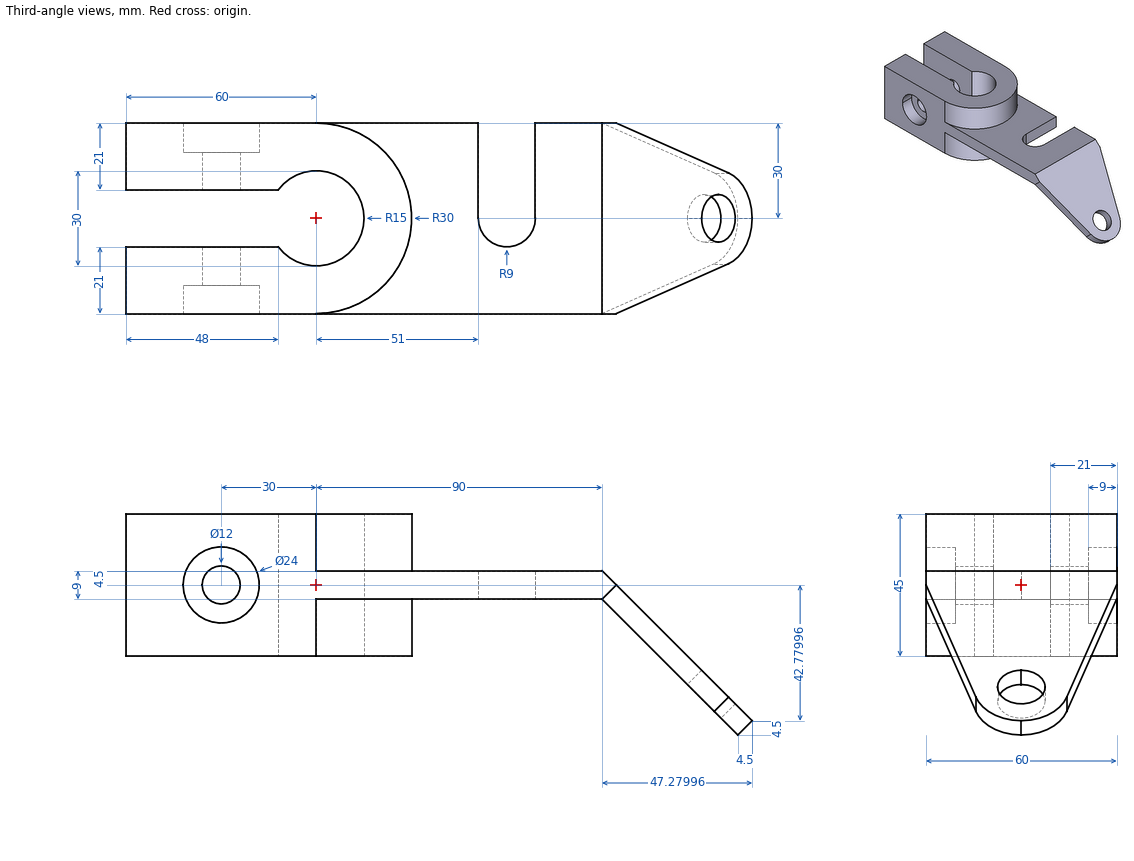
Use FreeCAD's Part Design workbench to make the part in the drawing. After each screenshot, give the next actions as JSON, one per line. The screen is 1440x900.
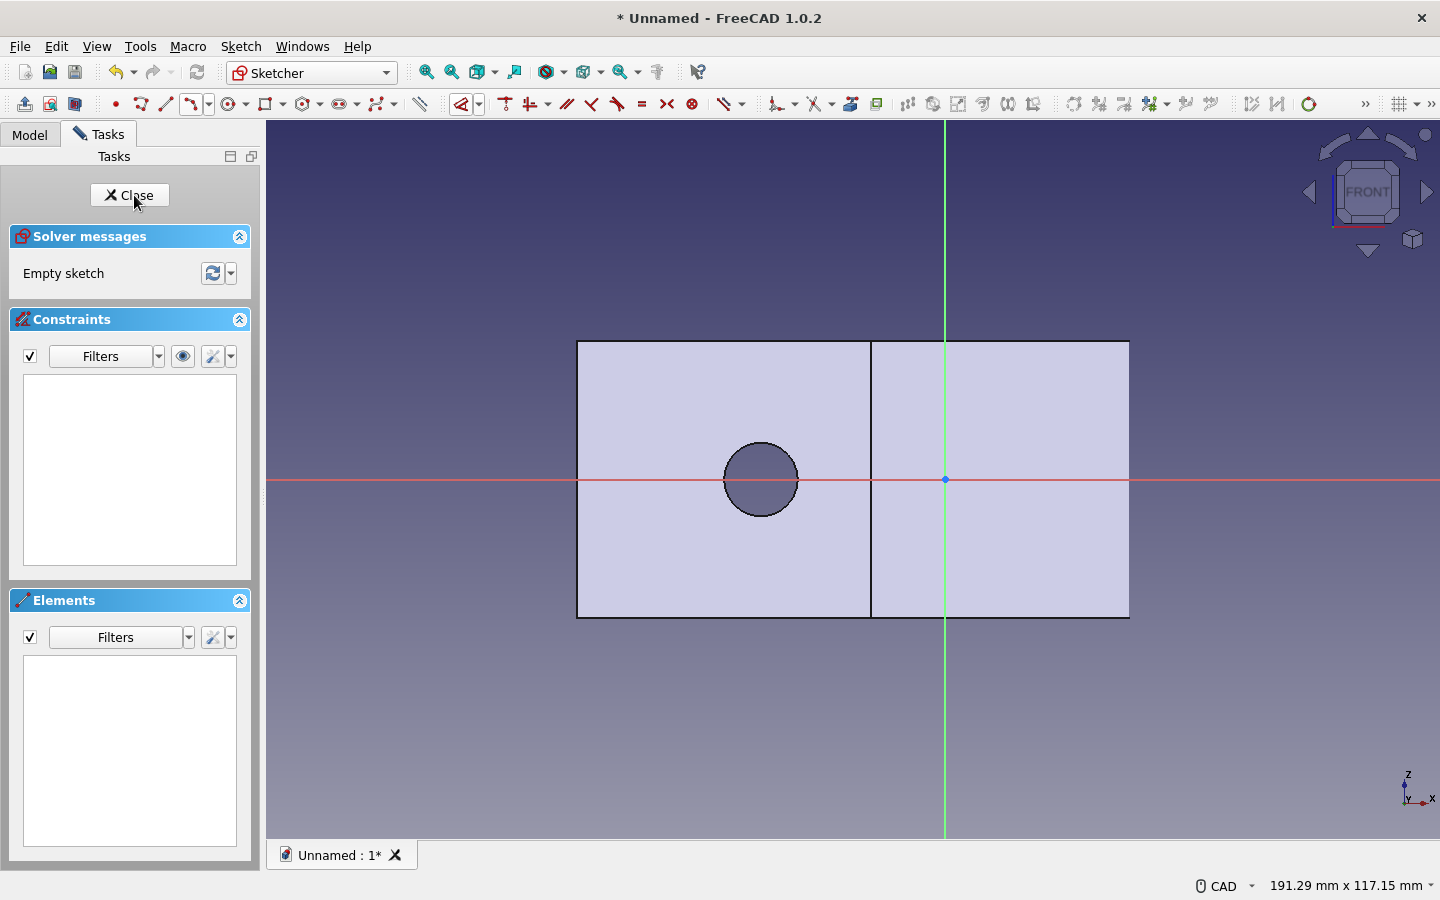
{"action": "scroll", "coordinate": [294, 320], "scroll_direction": "down", "scroll_amount": 3}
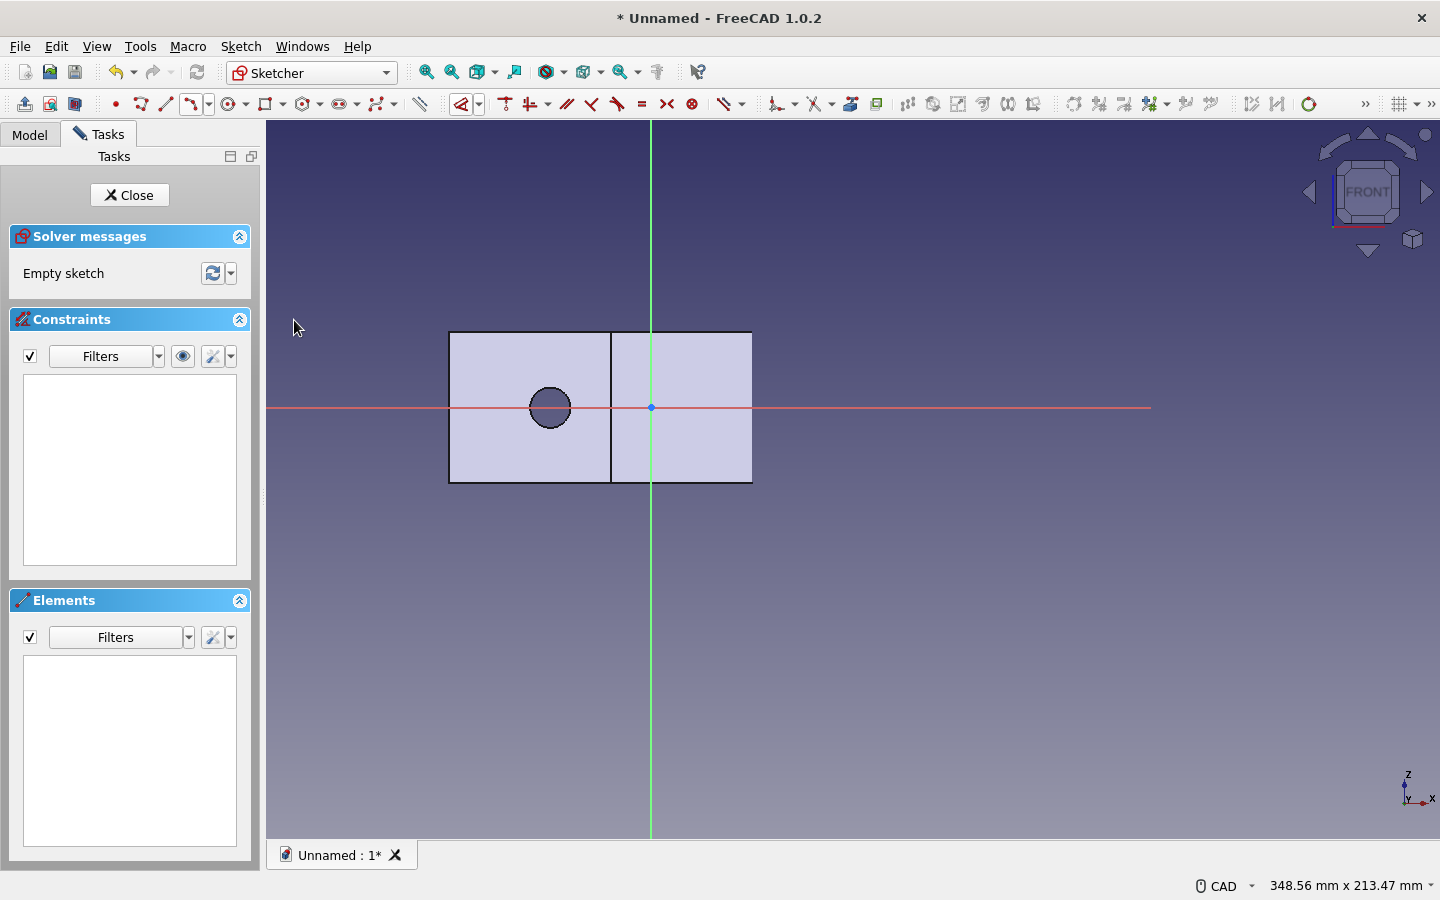
{"action": "scroll", "coordinate": [1082, 480], "scroll_direction": "up", "scroll_amount": 2}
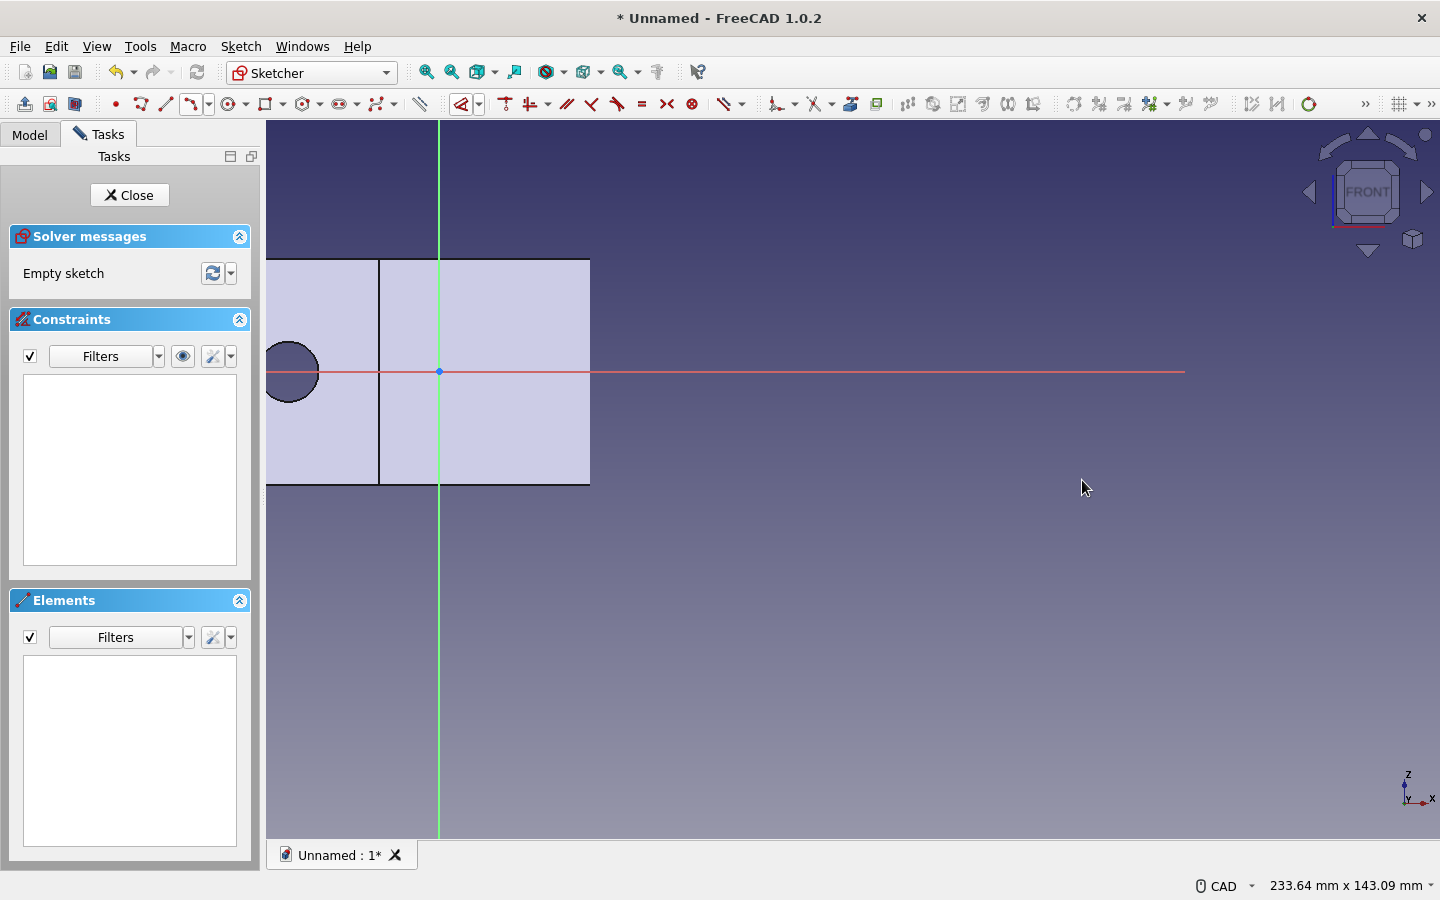
{"action": "left_click", "coordinate": [141, 104]}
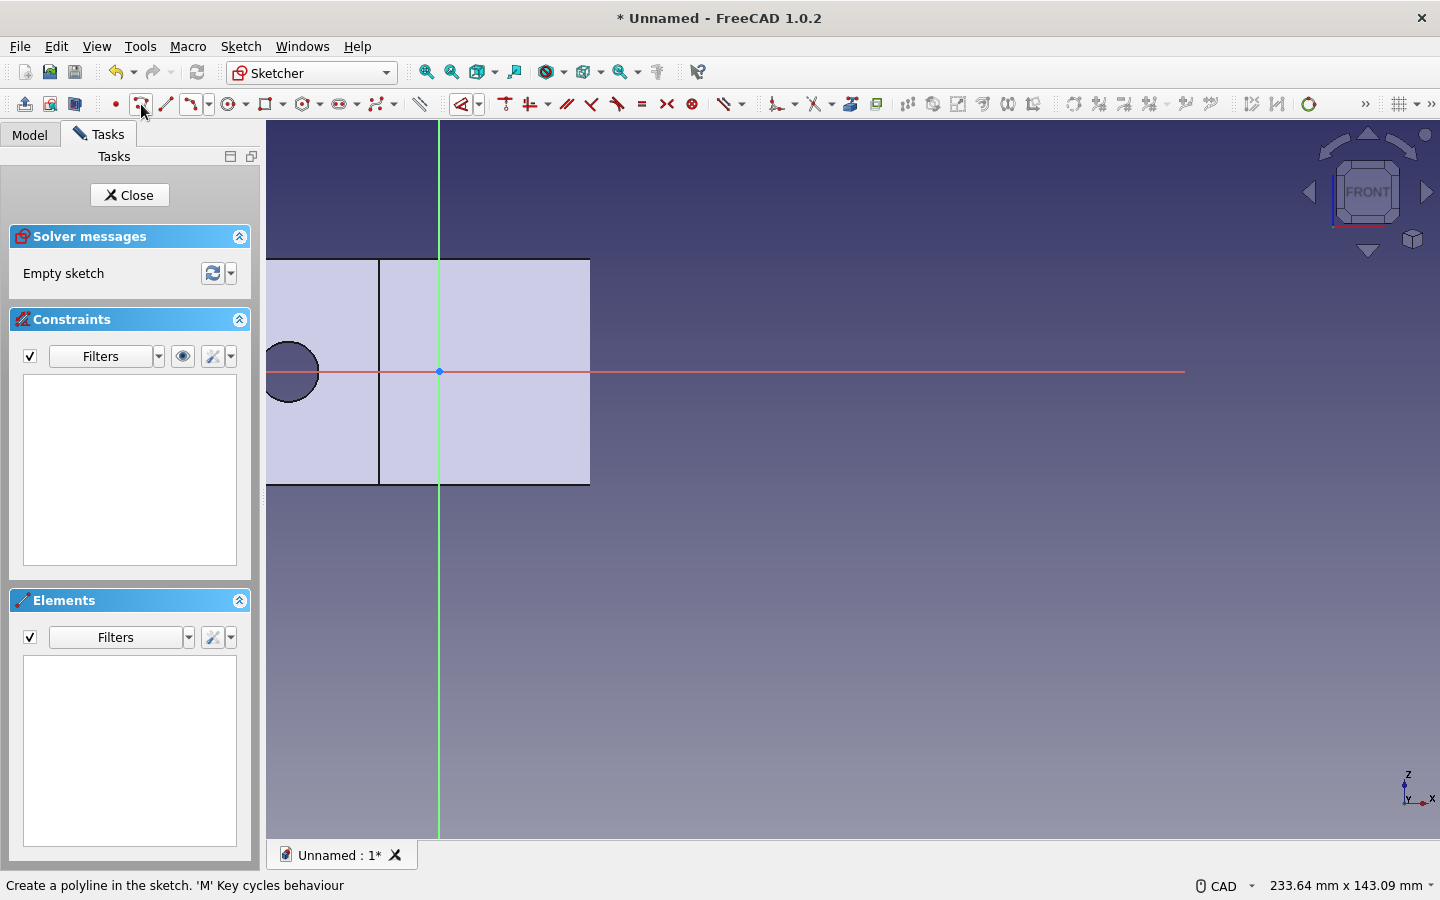
{"action": "left_click", "coordinate": [439, 349]}
{"action": "left_click", "coordinate": [891, 349]}
{"action": "left_click", "coordinate": [1129, 587]}
{"action": "left_click", "coordinate": [1106, 609]}
{"action": "left_click", "coordinate": [891, 394]}
{"action": "left_click", "coordinate": [448, 394]}
{"action": "left_click", "coordinate": [439, 350]}
{"action": "key", "text": "Escape"}
{"action": "key", "text": "Escape"}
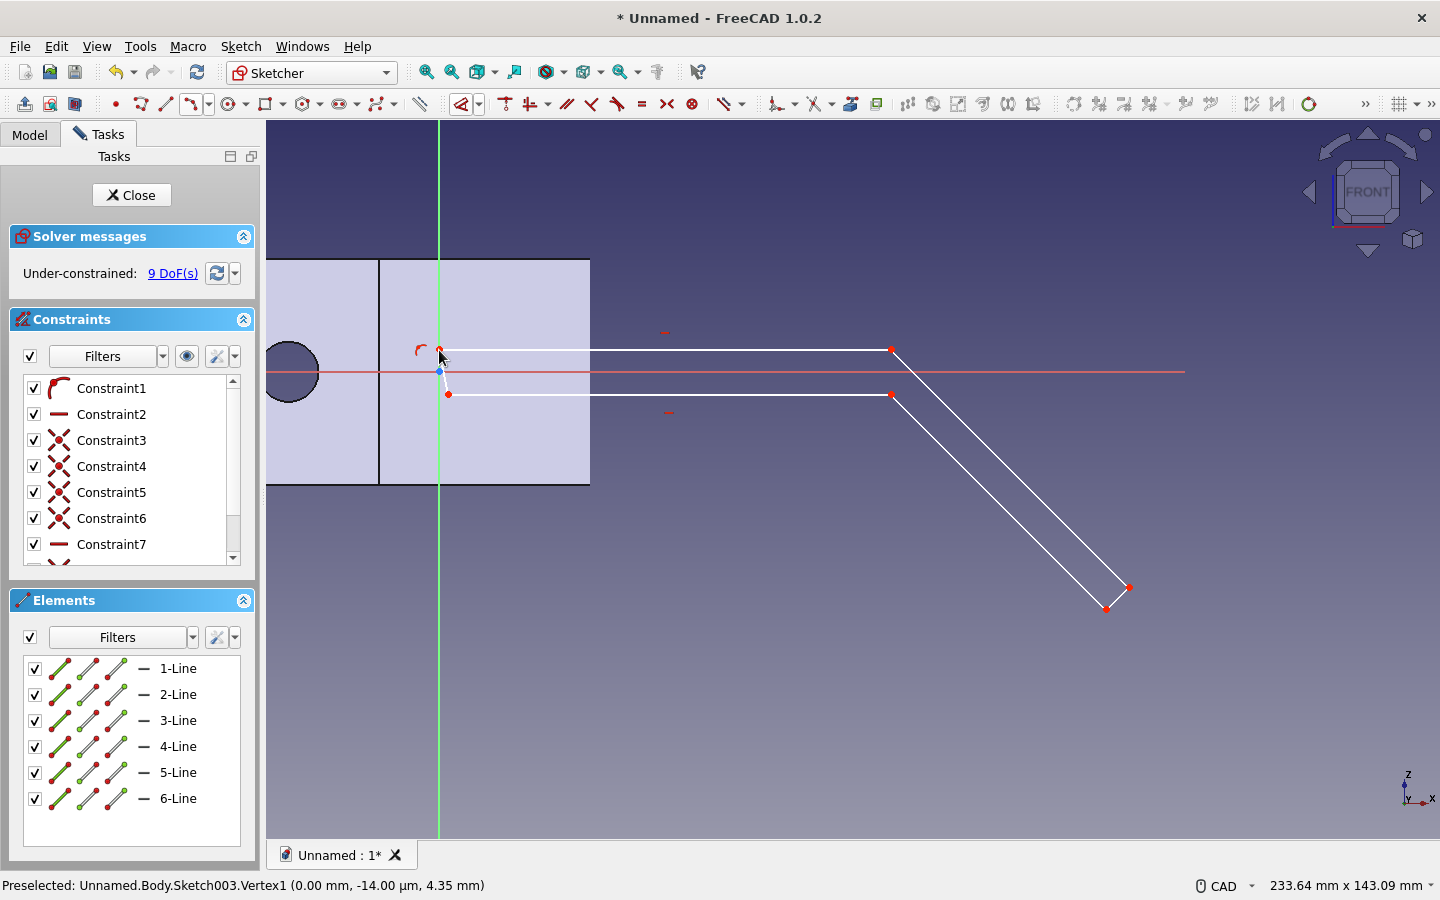
{"action": "left_click", "coordinate": [441, 359]}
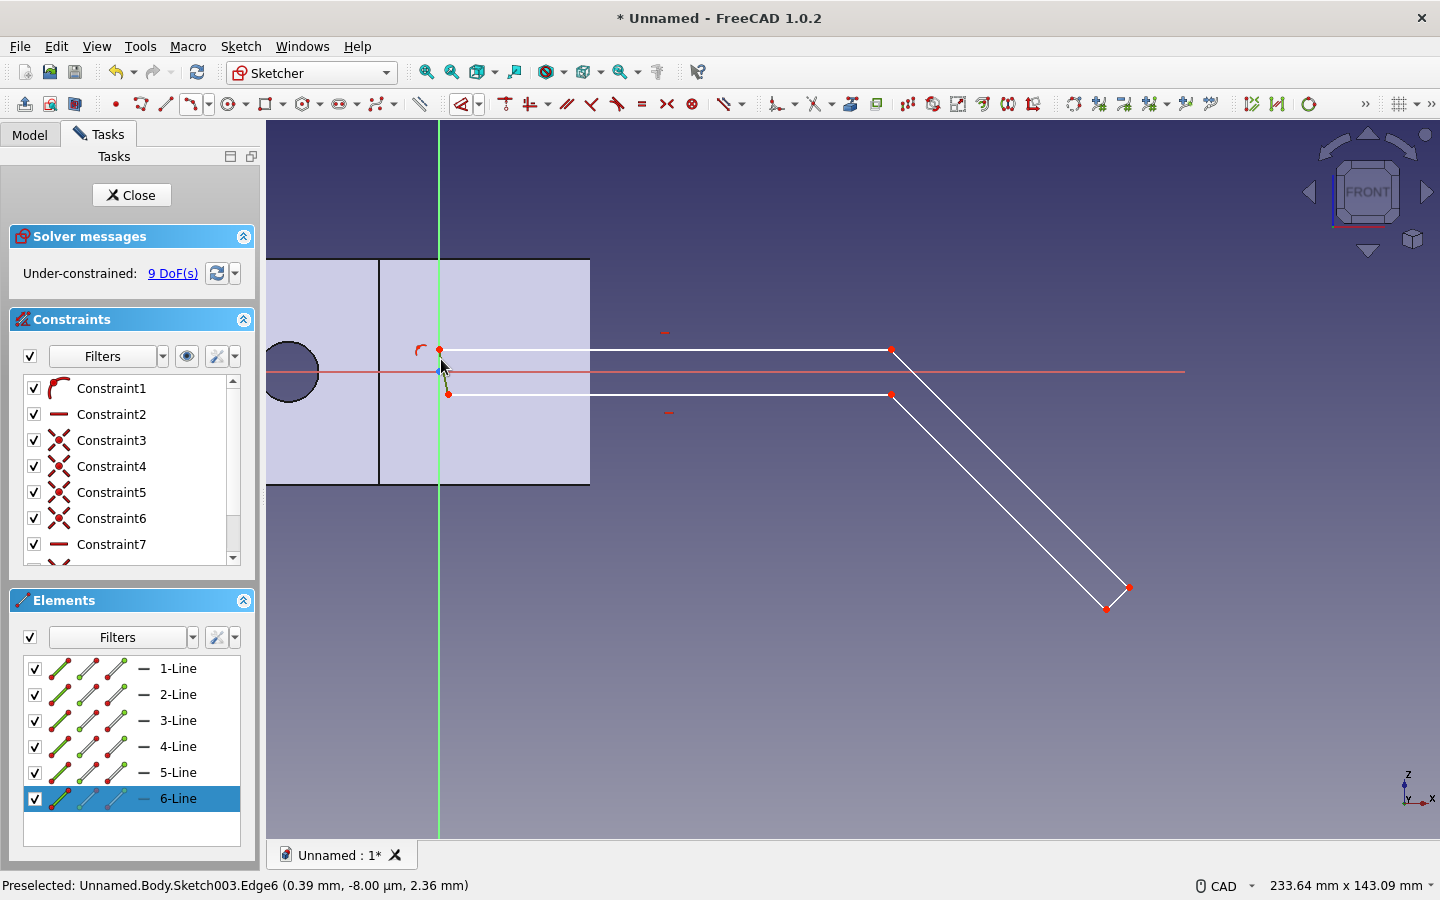
{"action": "left_click", "coordinate": [548, 104]}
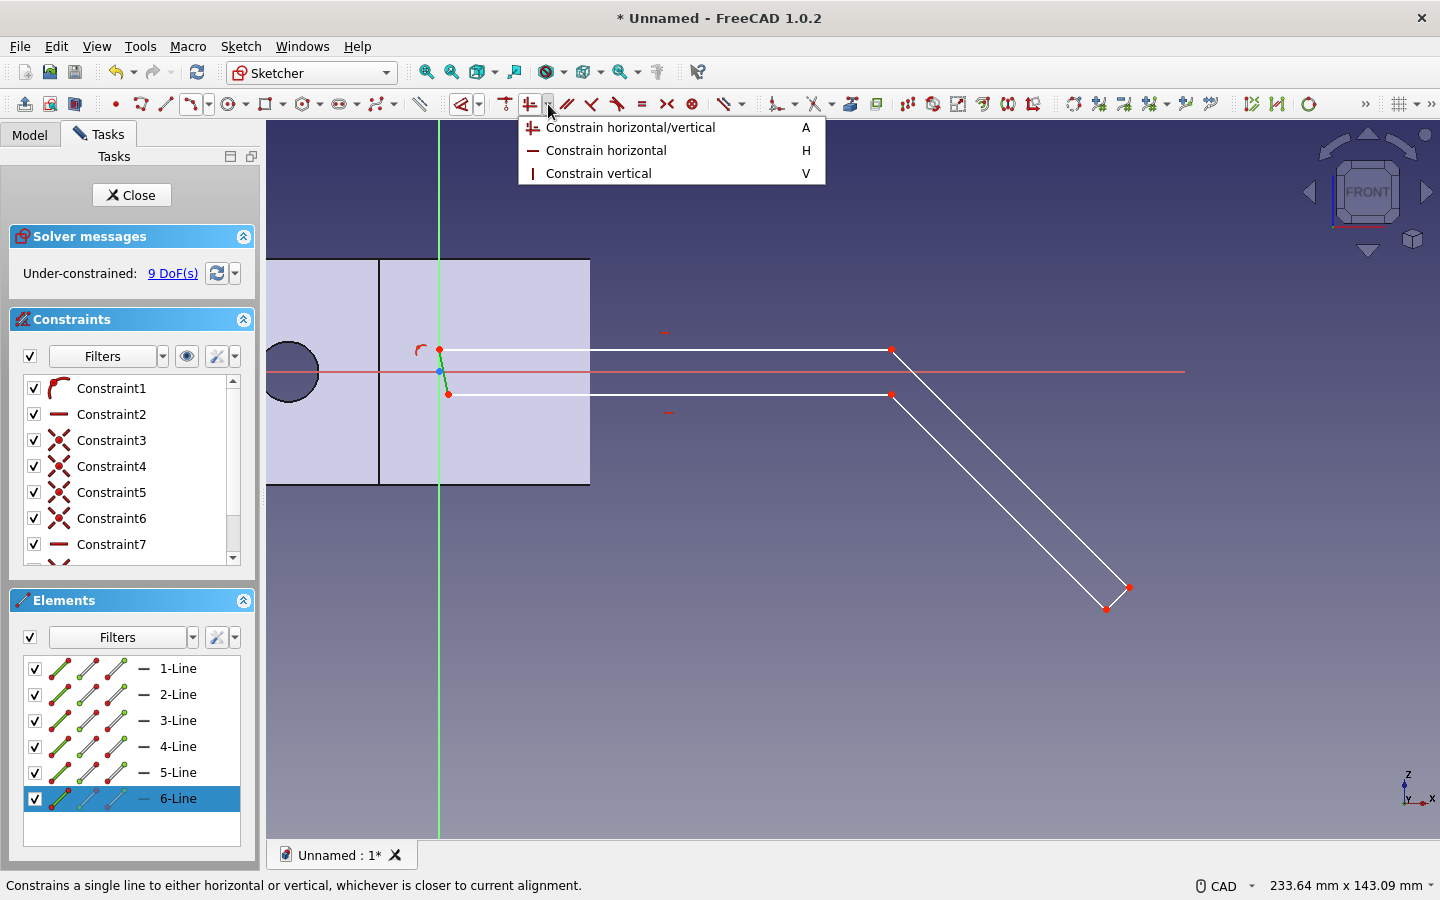
{"action": "left_click", "coordinate": [672, 174]}